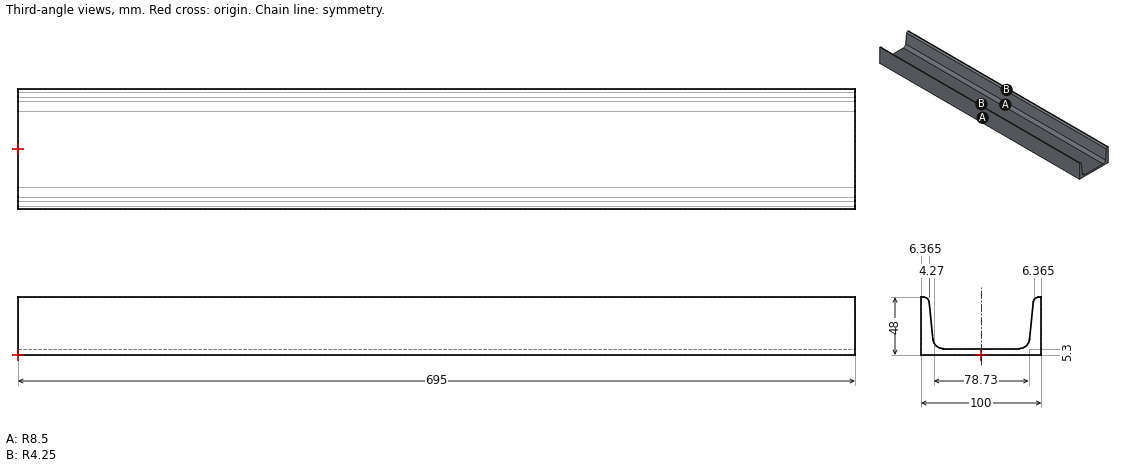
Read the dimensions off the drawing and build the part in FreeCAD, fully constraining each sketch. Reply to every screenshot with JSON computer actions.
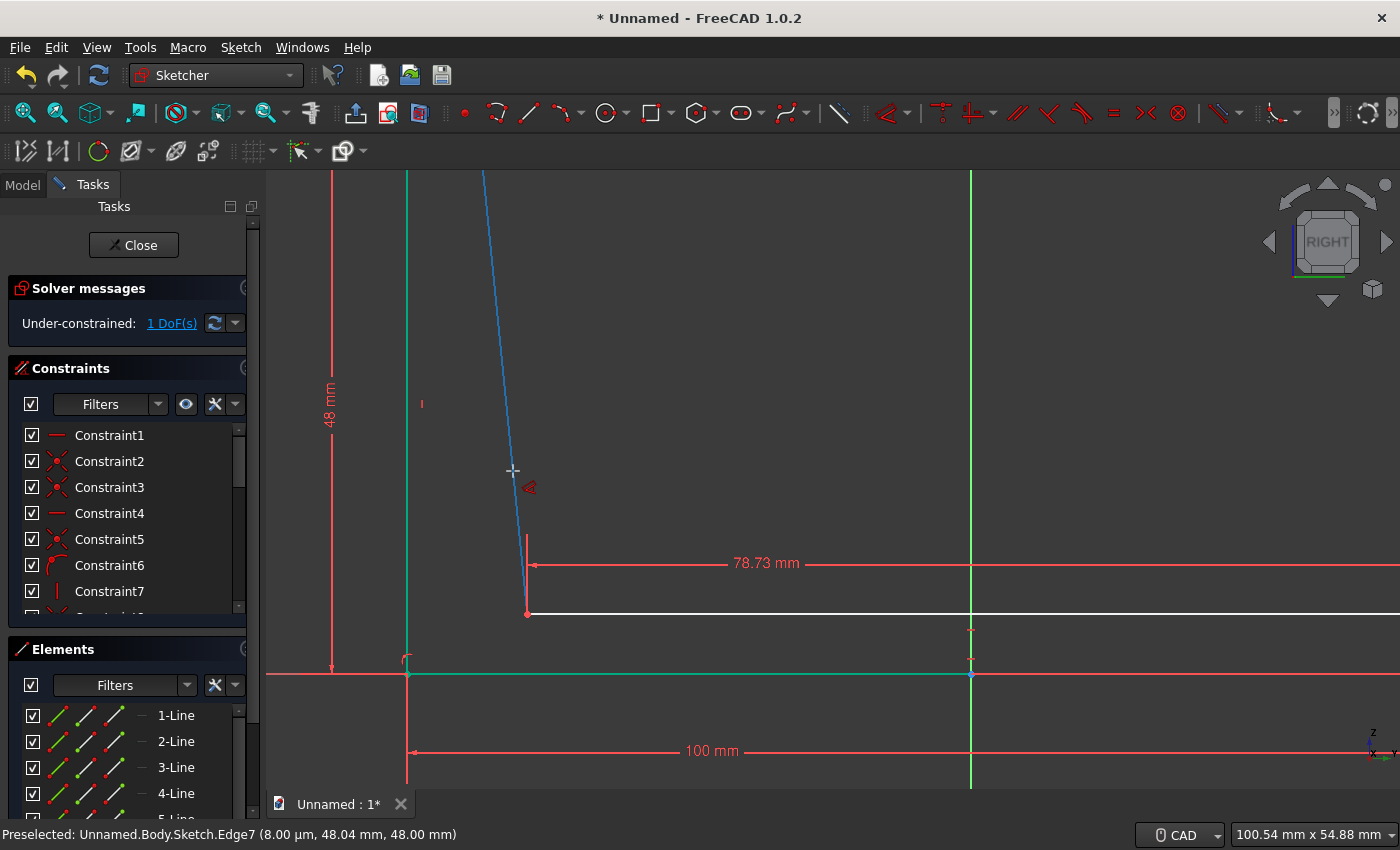
{"action": "left_click", "coordinate": [513, 470]}
{"action": "left_click", "coordinate": [503, 648]}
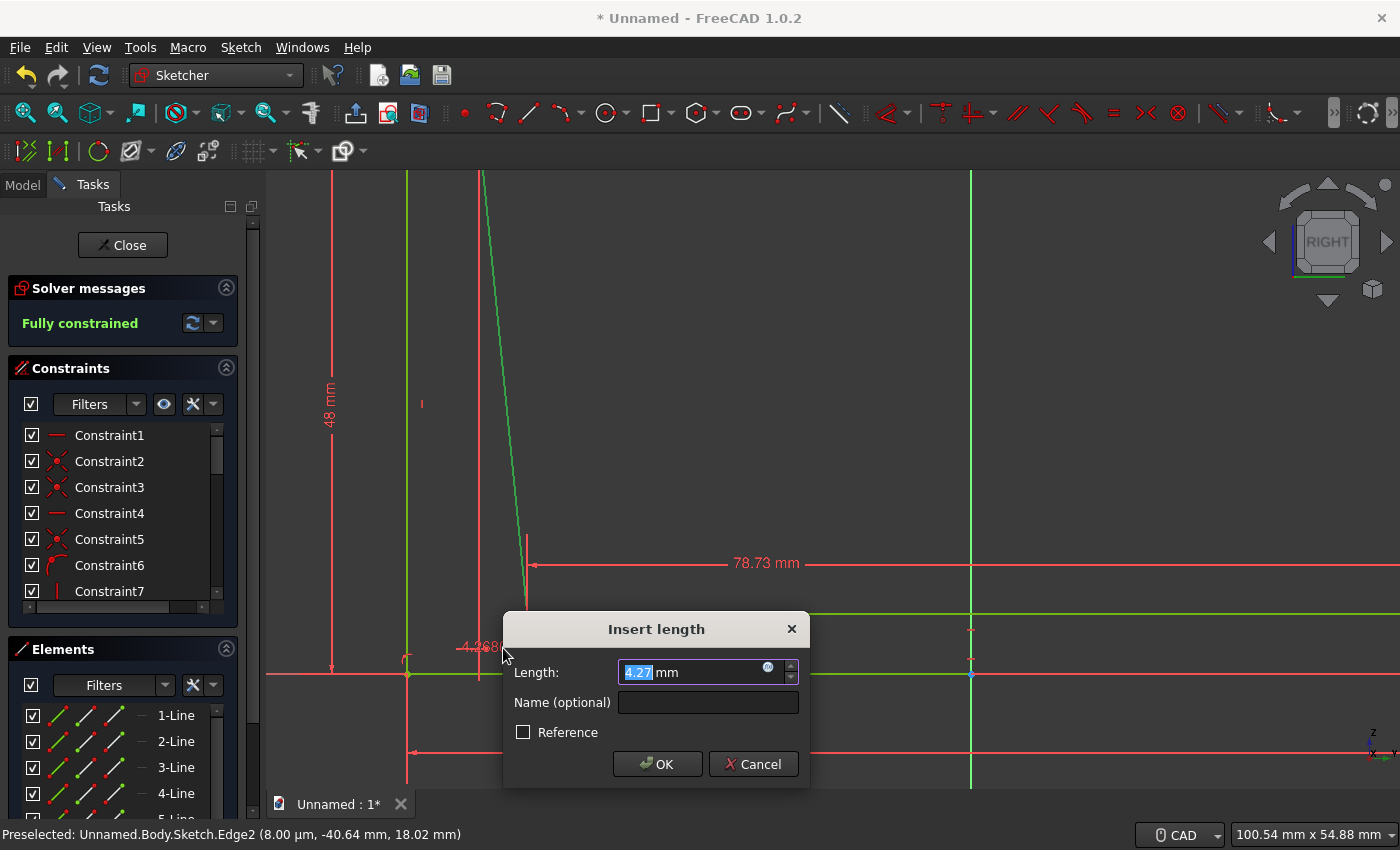
{"action": "type", "text": "4.27"}
{"action": "key", "text": "Return"}
{"action": "key", "text": "Escape"}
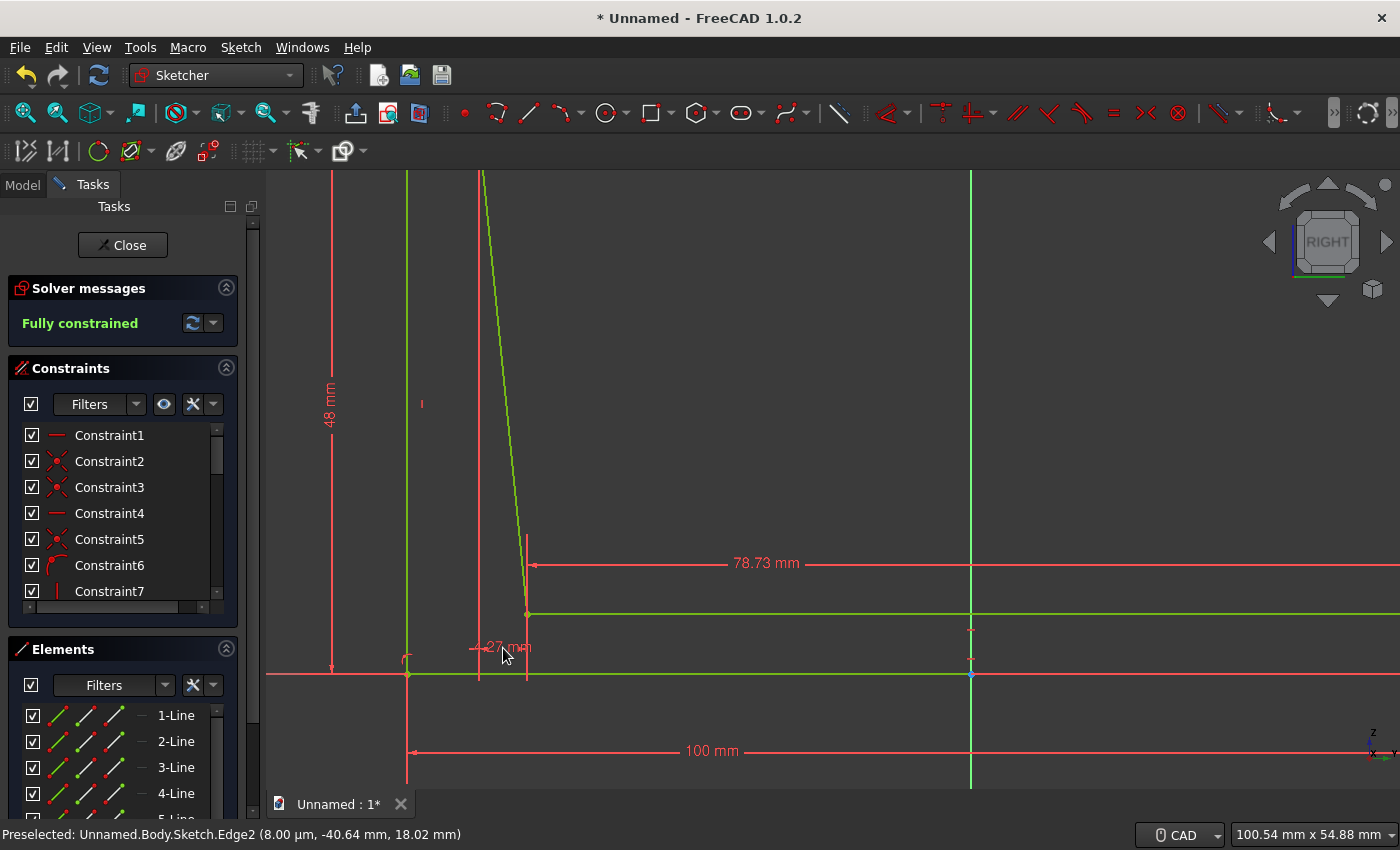
{"action": "left_click", "coordinate": [123, 245]}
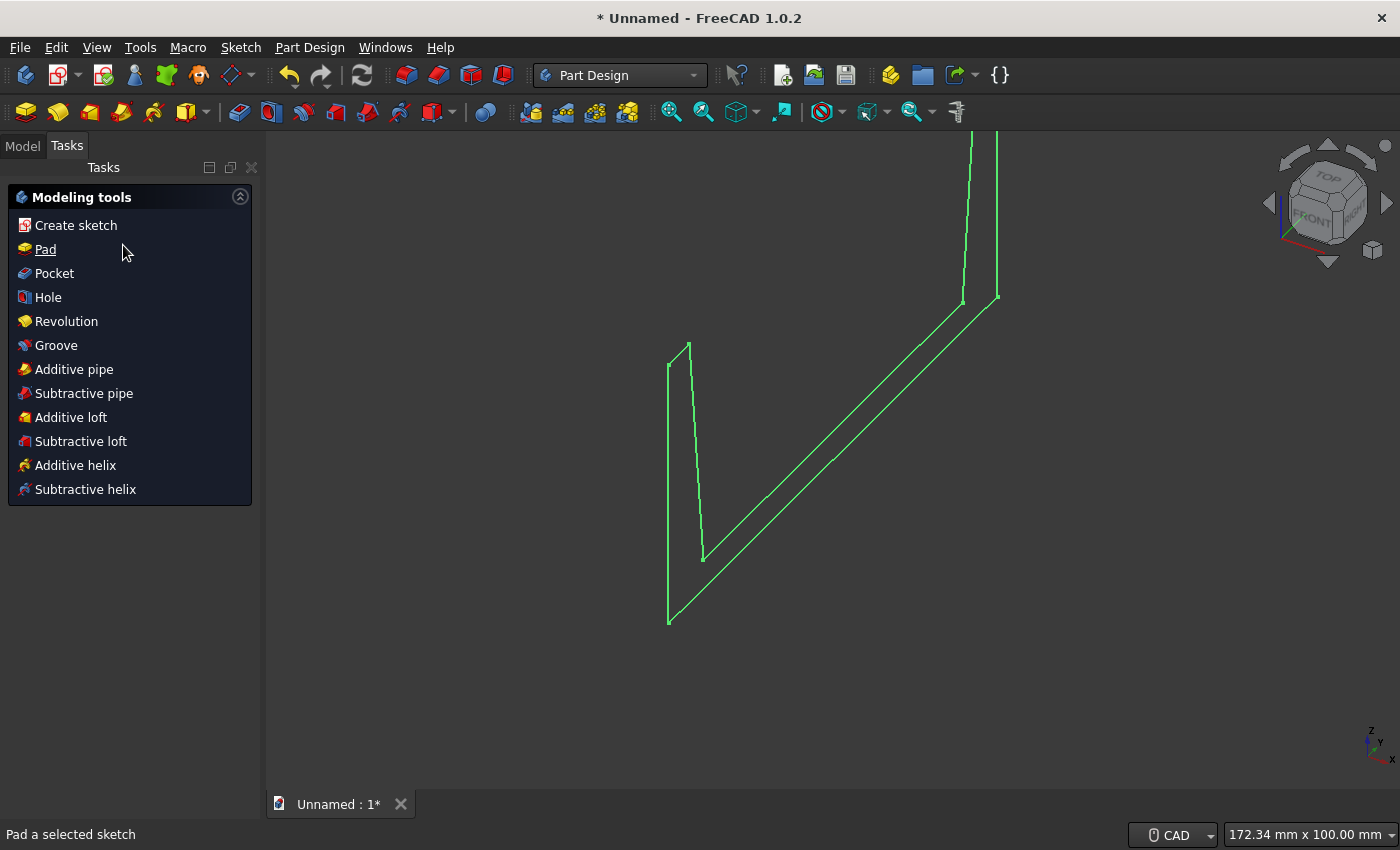
{"action": "left_click", "coordinate": [26, 112]}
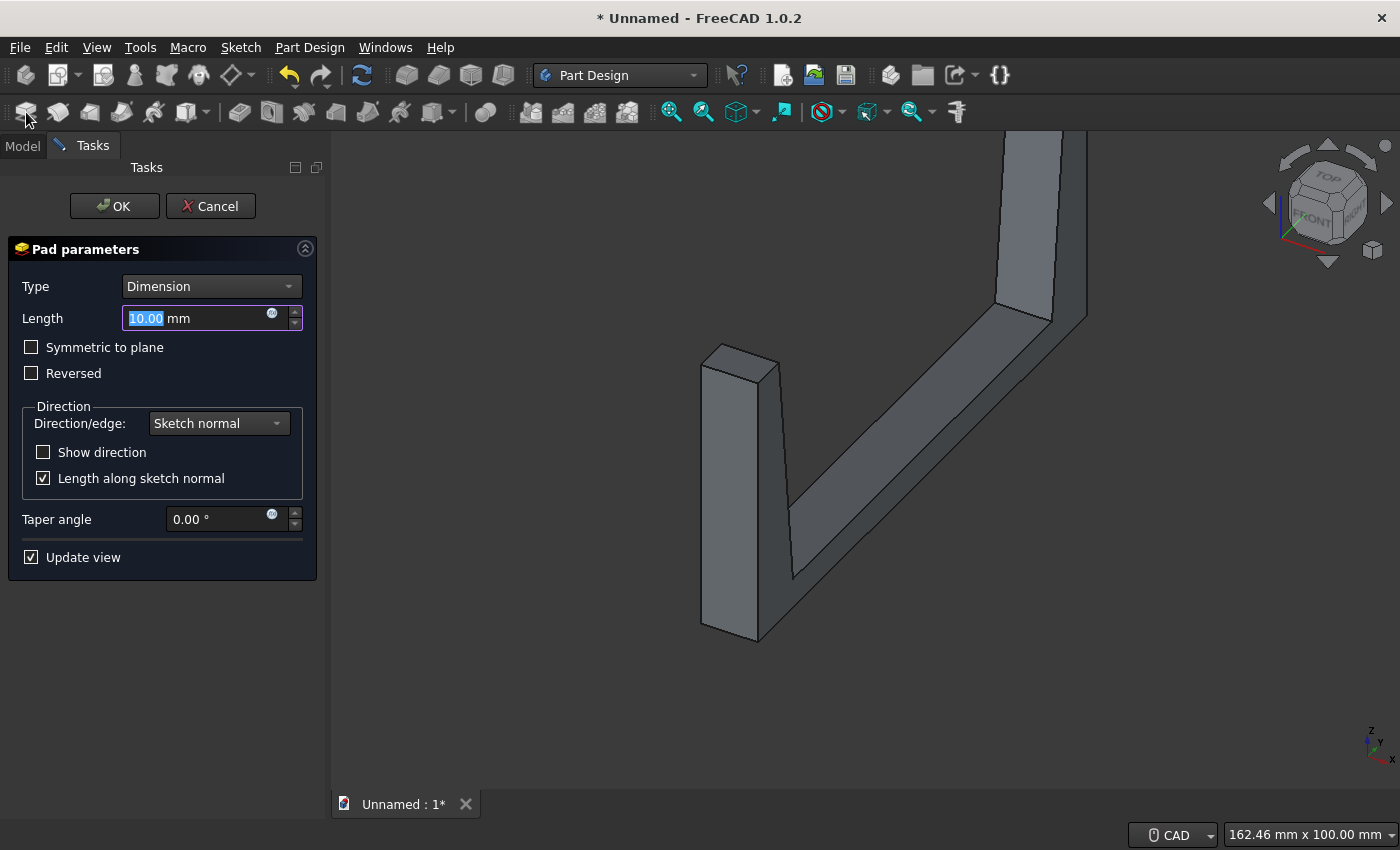
{"action": "type", "text": "695"}
{"action": "key", "text": "Tab"}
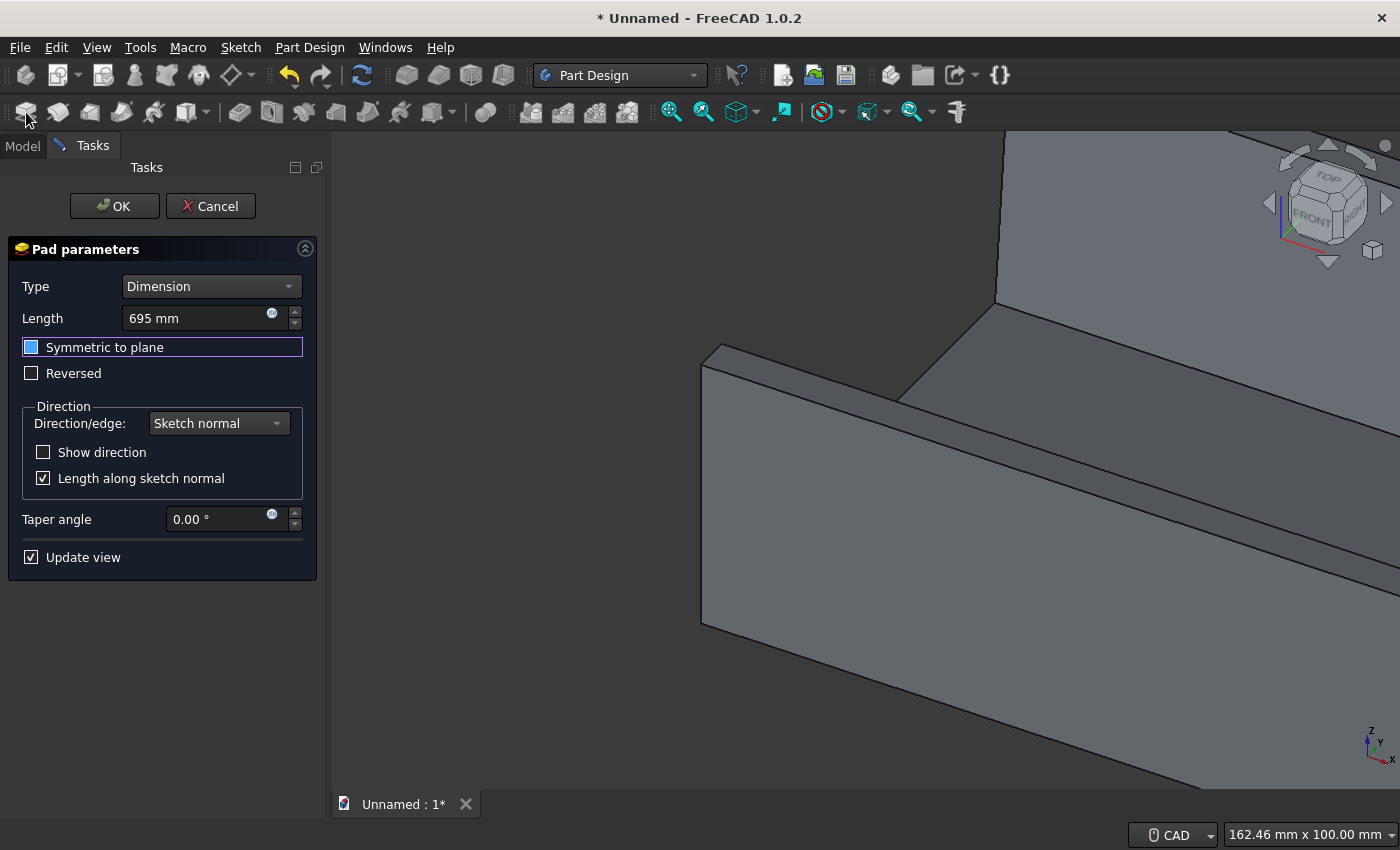
{"action": "left_click", "coordinate": [115, 206]}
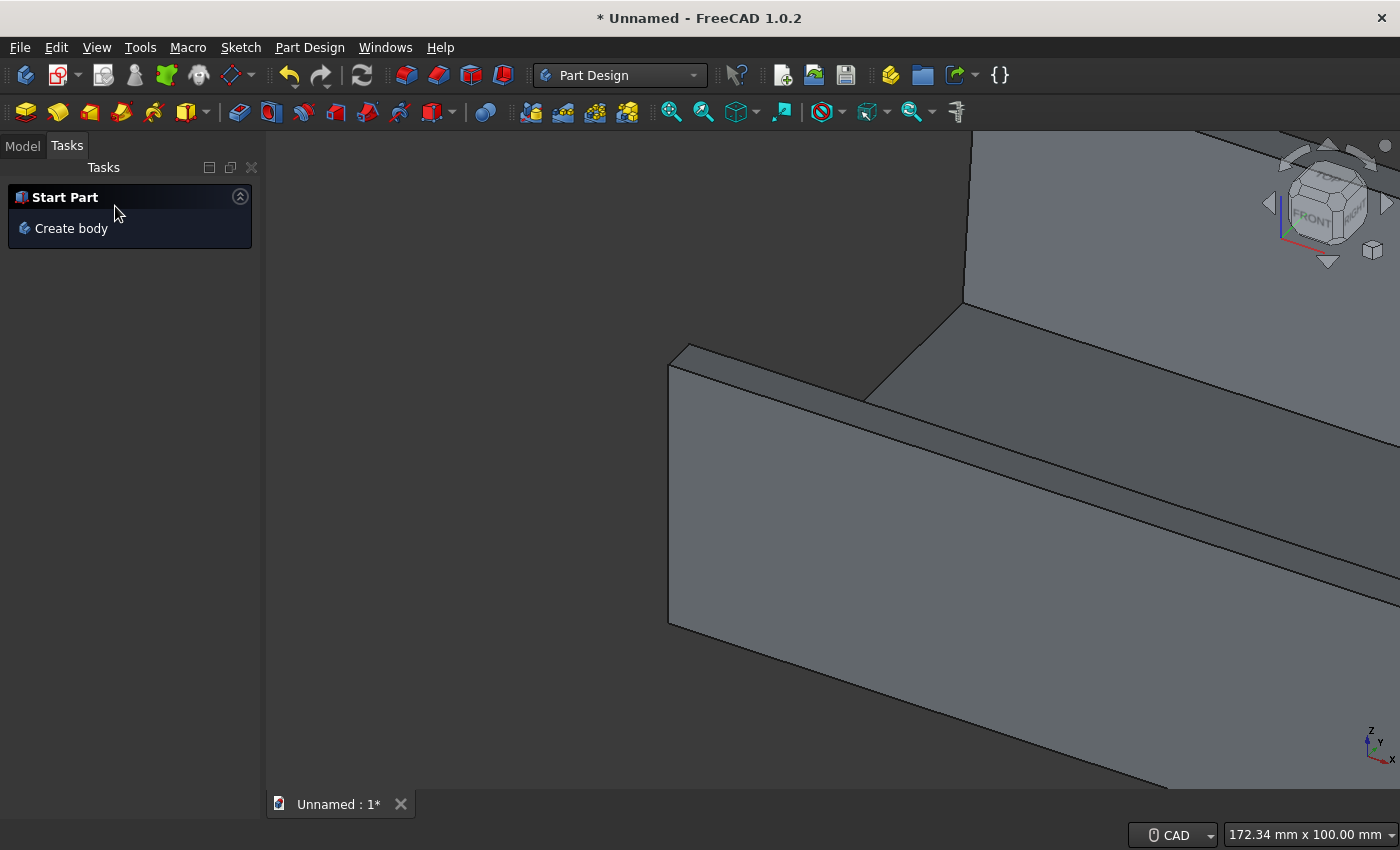
{"action": "left_click", "coordinate": [672, 112]}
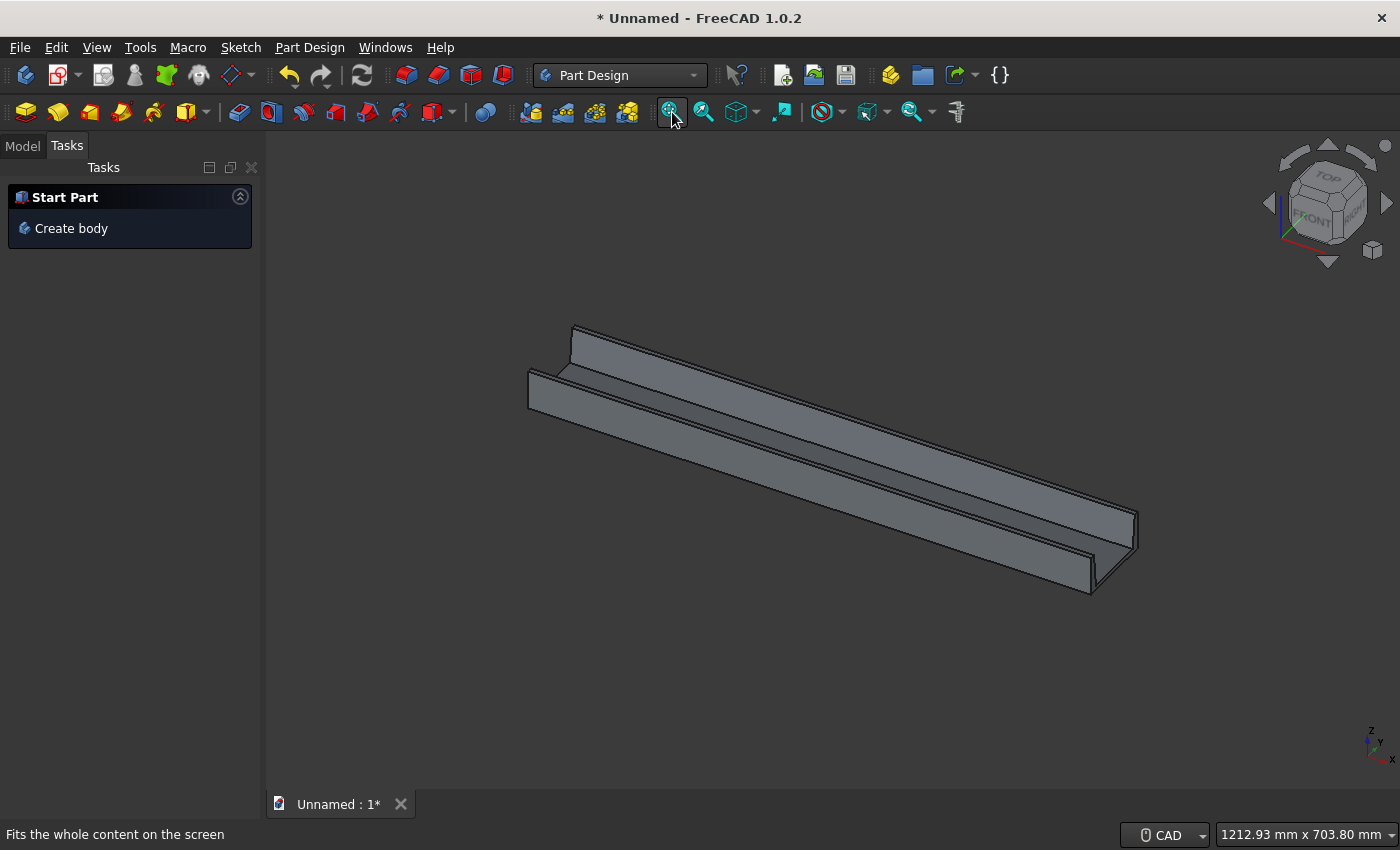
{"action": "key", "text": "0"}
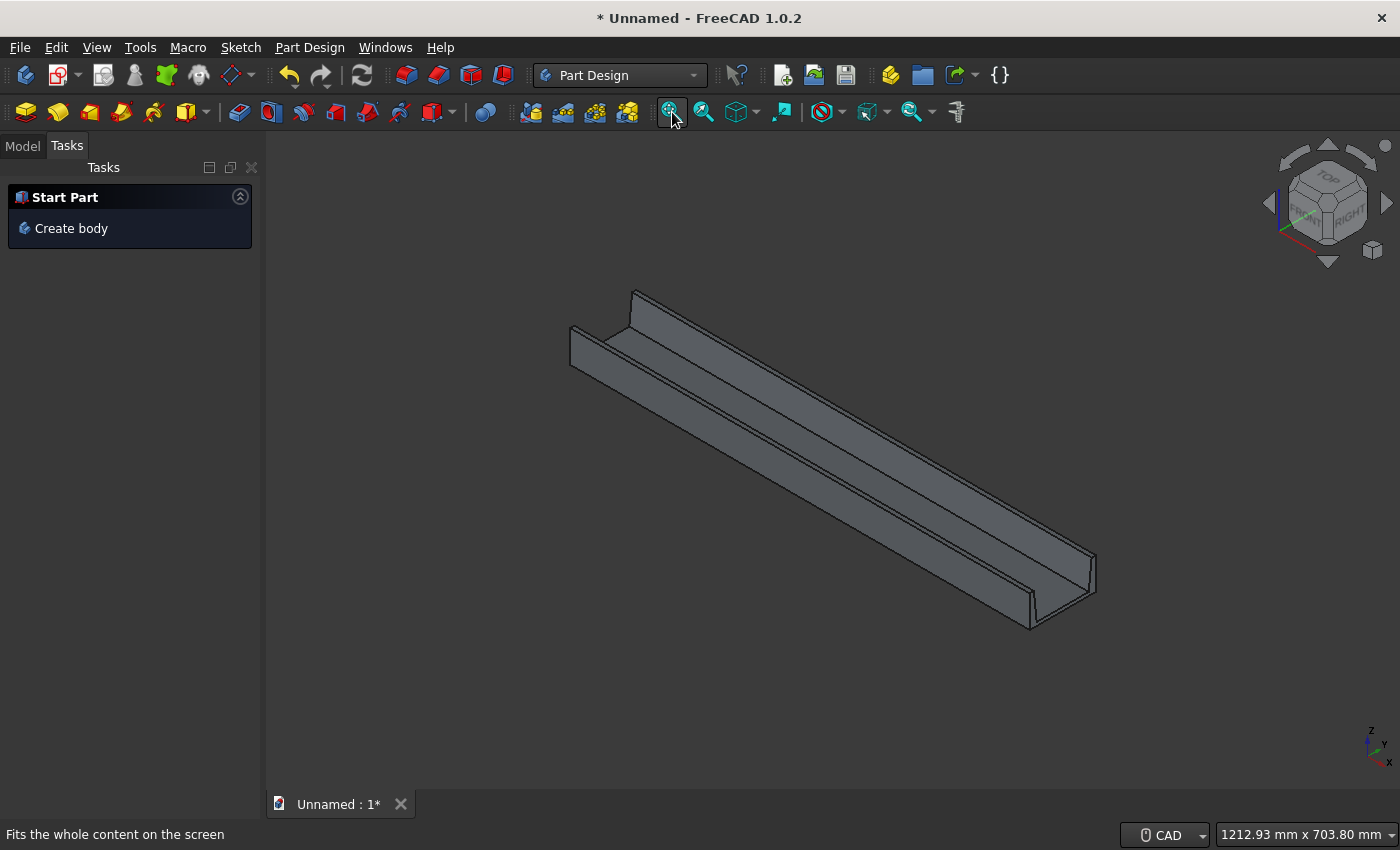
{"action": "key", "text": "2"}